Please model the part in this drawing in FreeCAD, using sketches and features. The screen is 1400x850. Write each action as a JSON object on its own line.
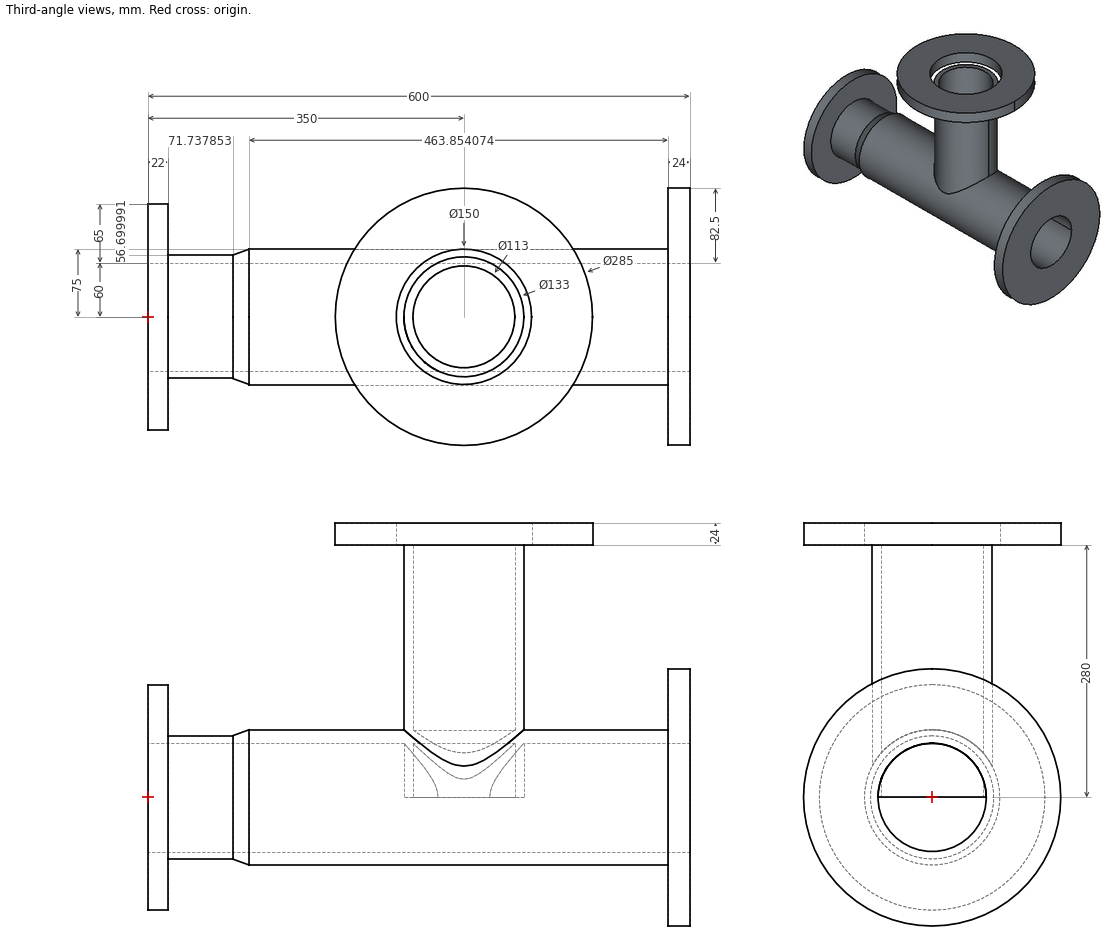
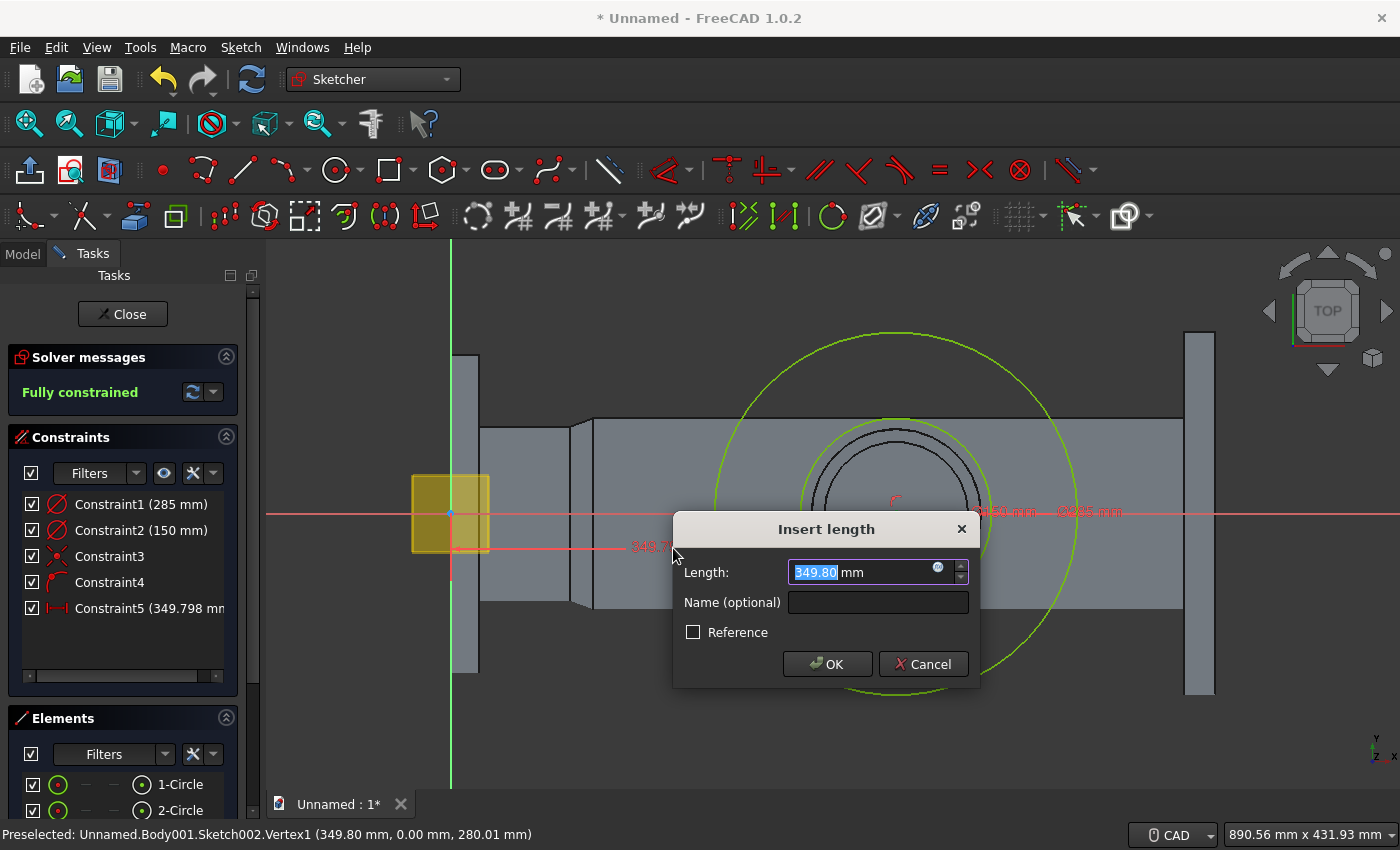
{"action": "type", "text": "350"}
{"action": "key", "text": "Return"}
{"action": "key", "text": "Escape"}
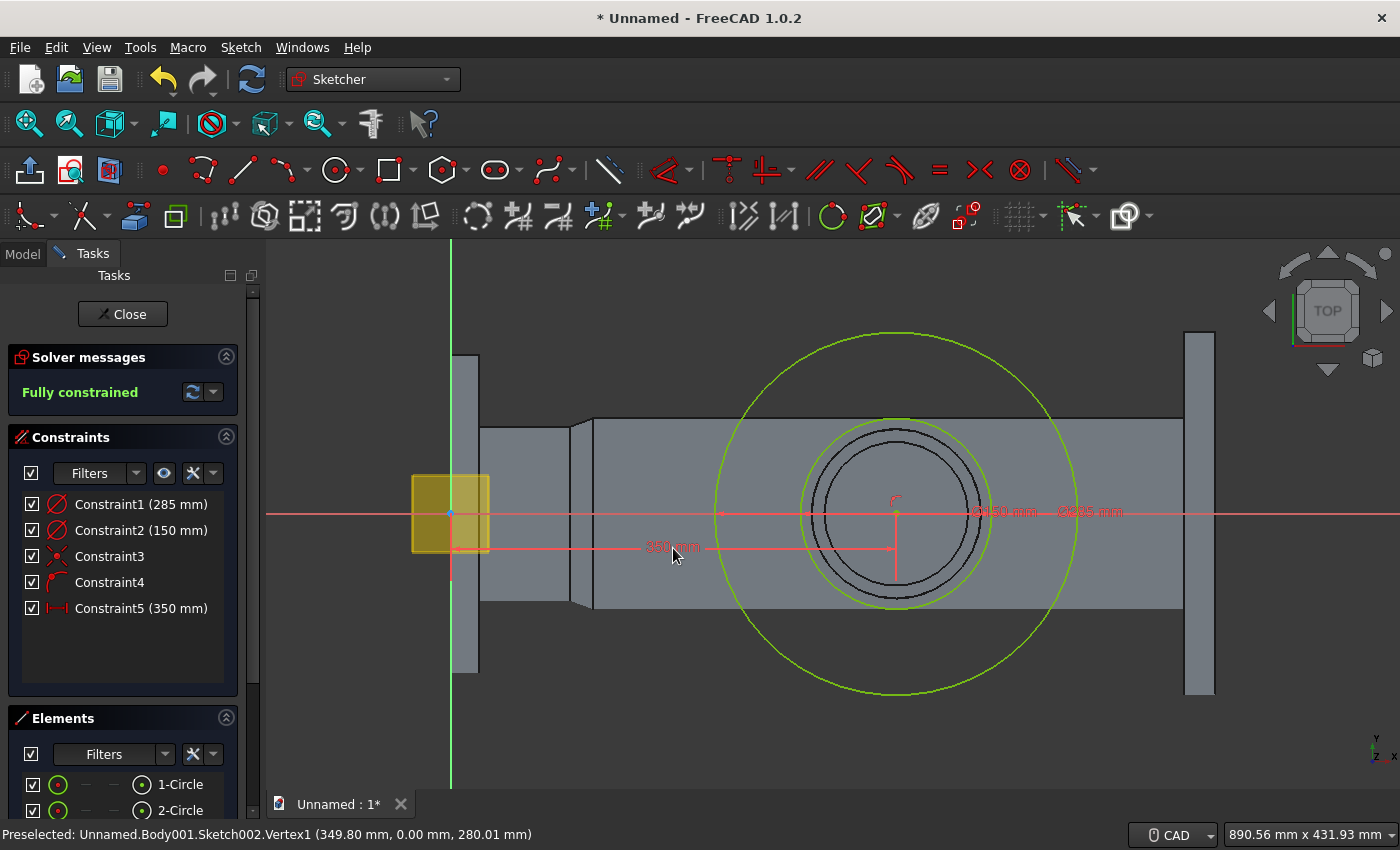
{"action": "left_click", "coordinate": [123, 314]}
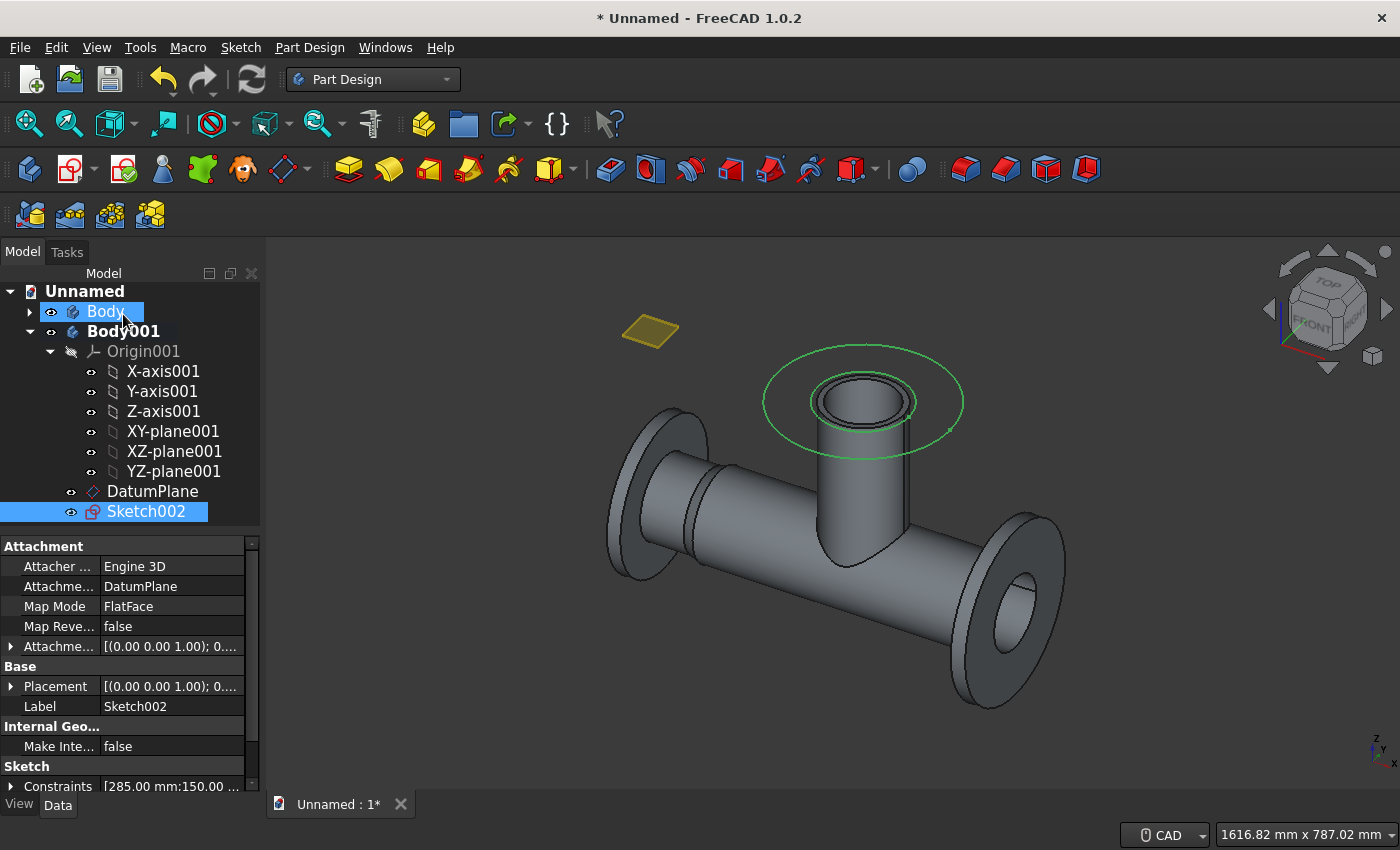
{"action": "left_click", "coordinate": [350, 170]}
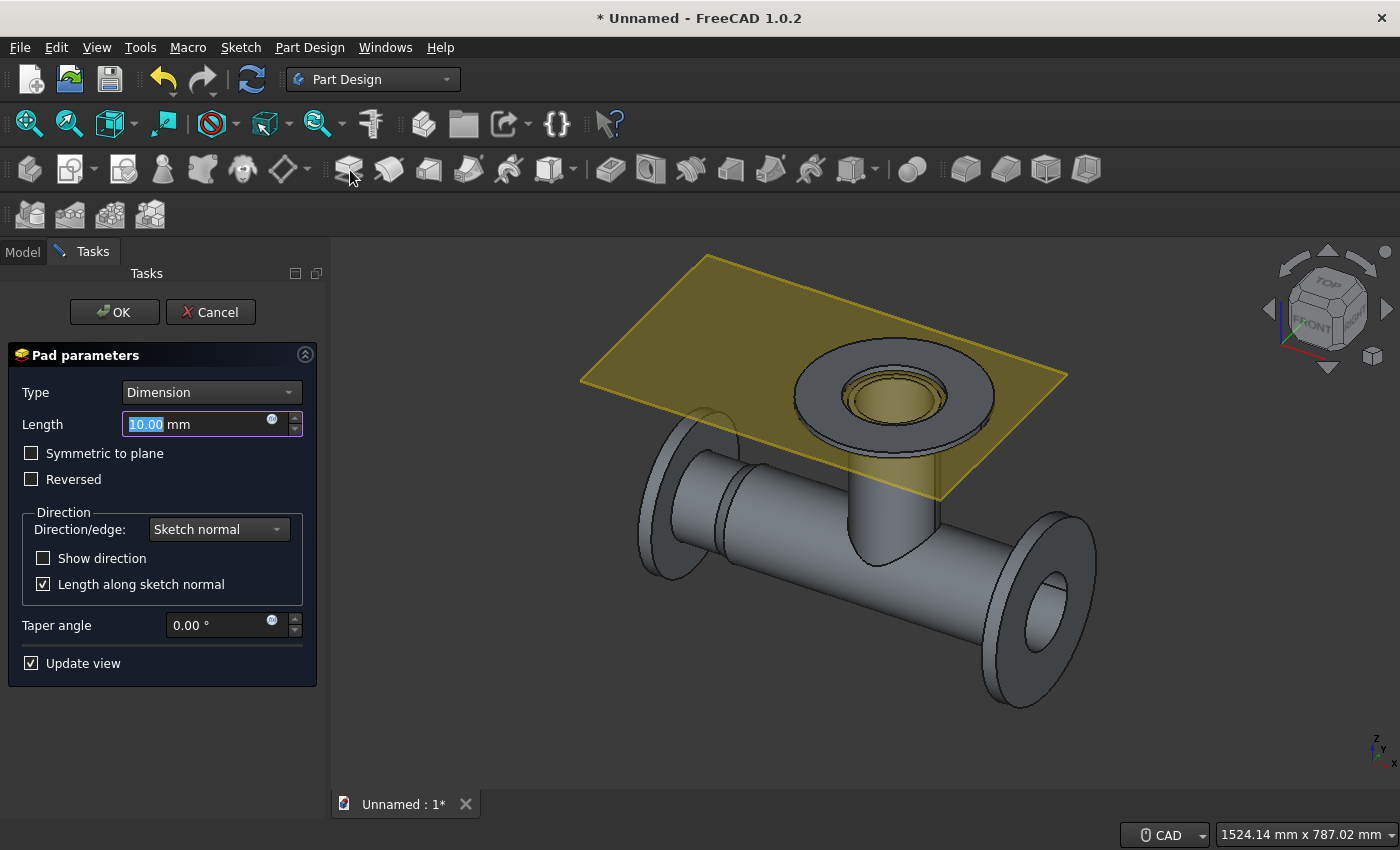
{"action": "type", "text": "24"}
{"action": "key", "text": "Tab"}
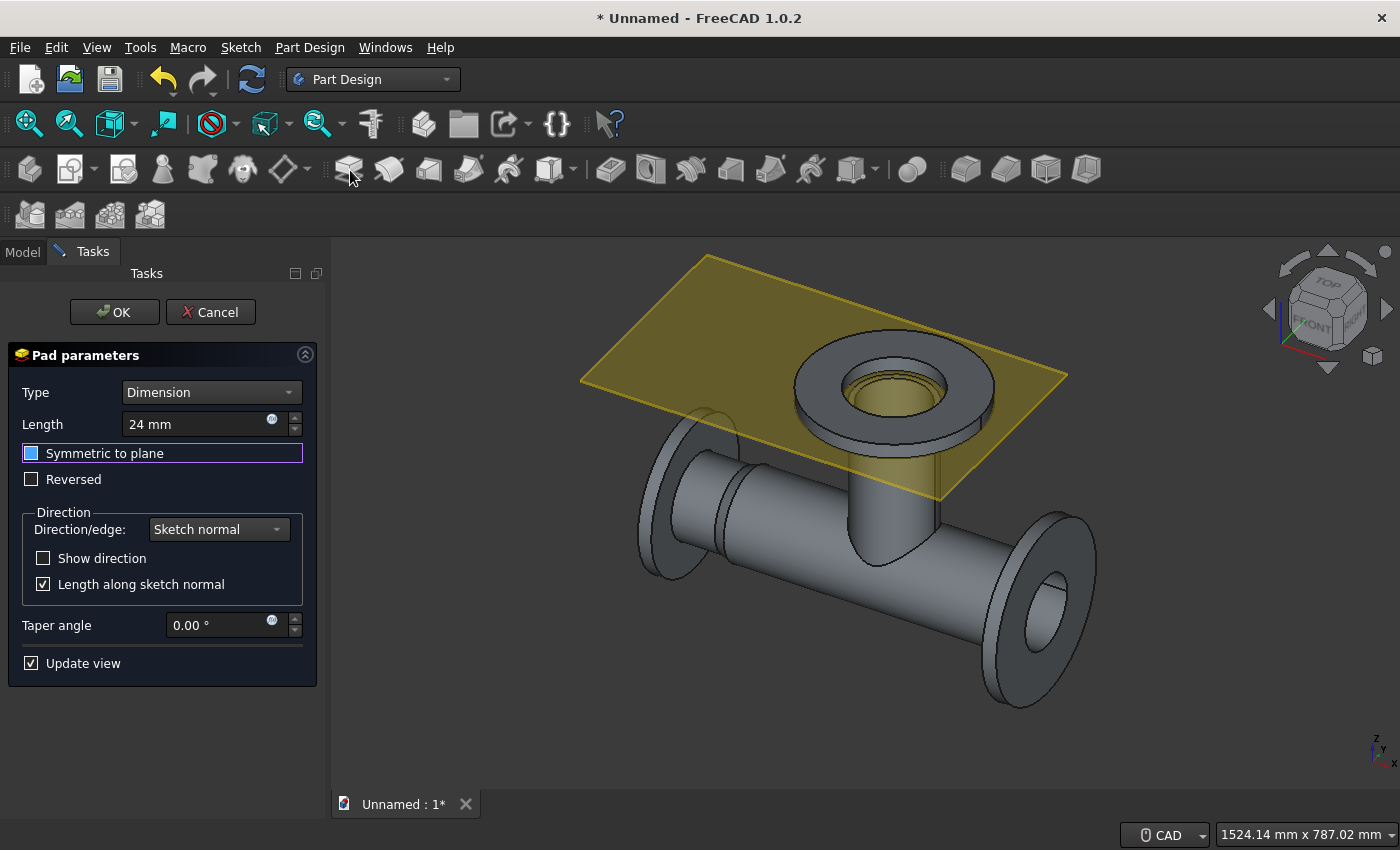
{"action": "left_click", "coordinate": [115, 312]}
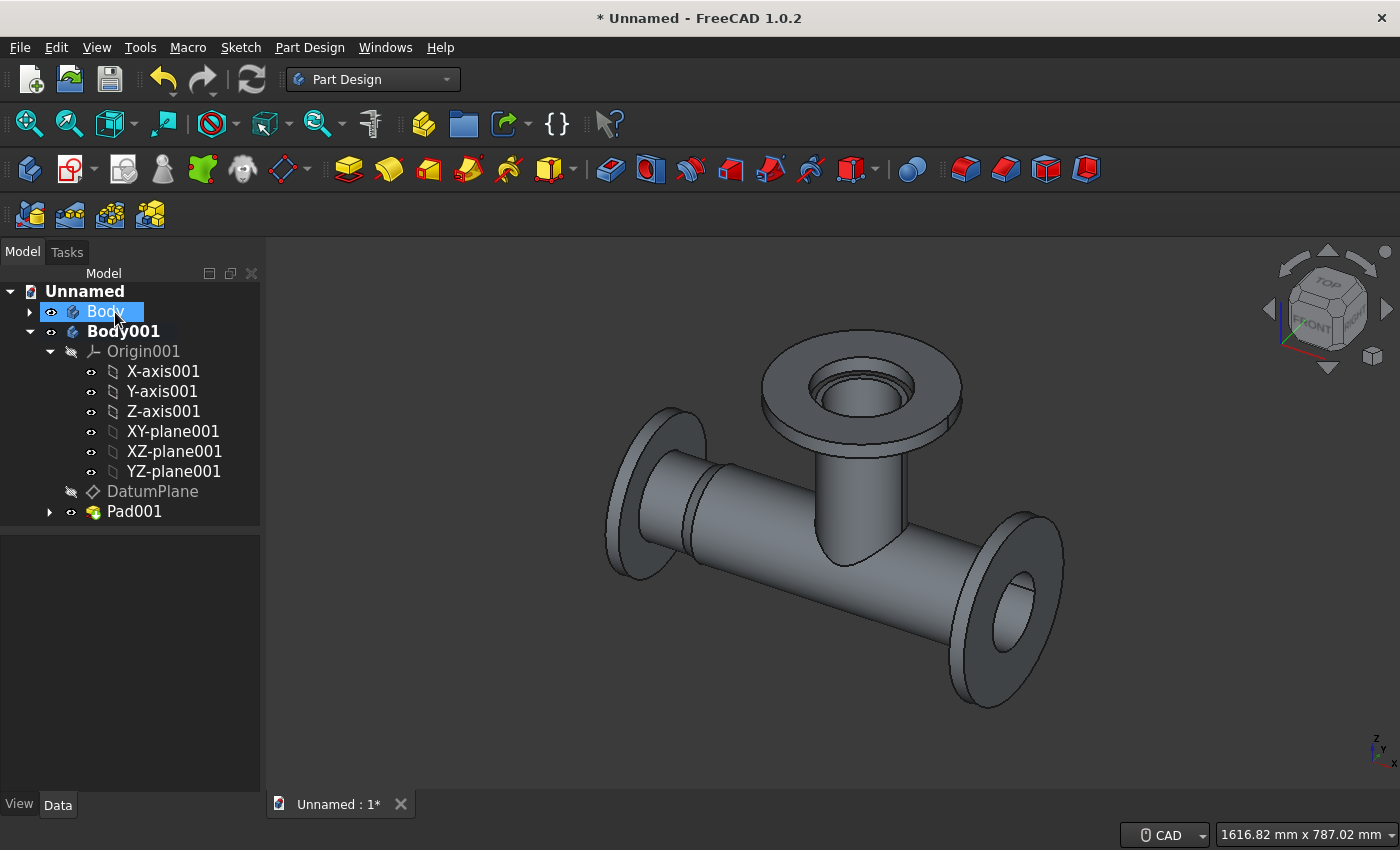
{"action": "key", "text": "0"}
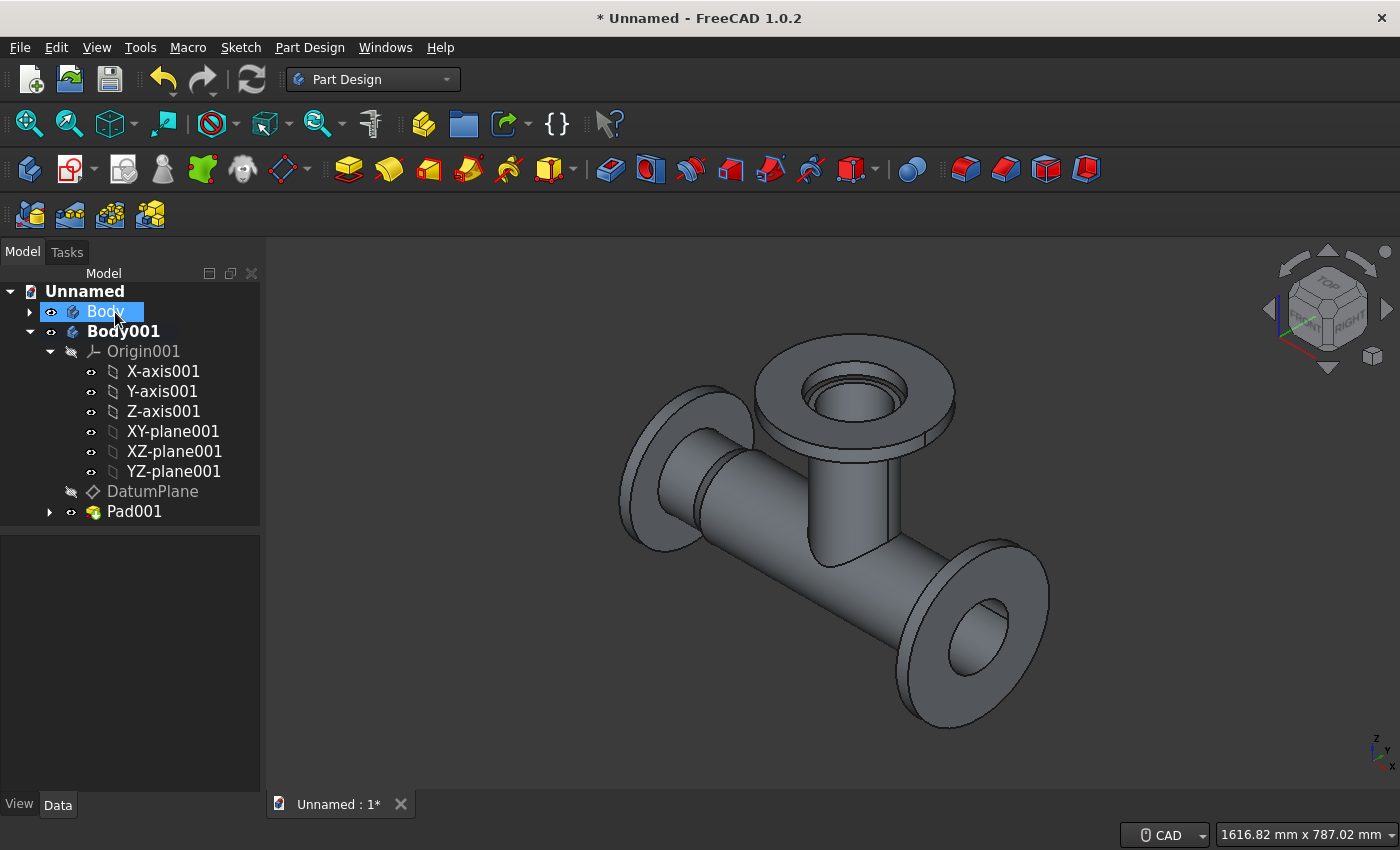
{"action": "key", "text": "v f"}